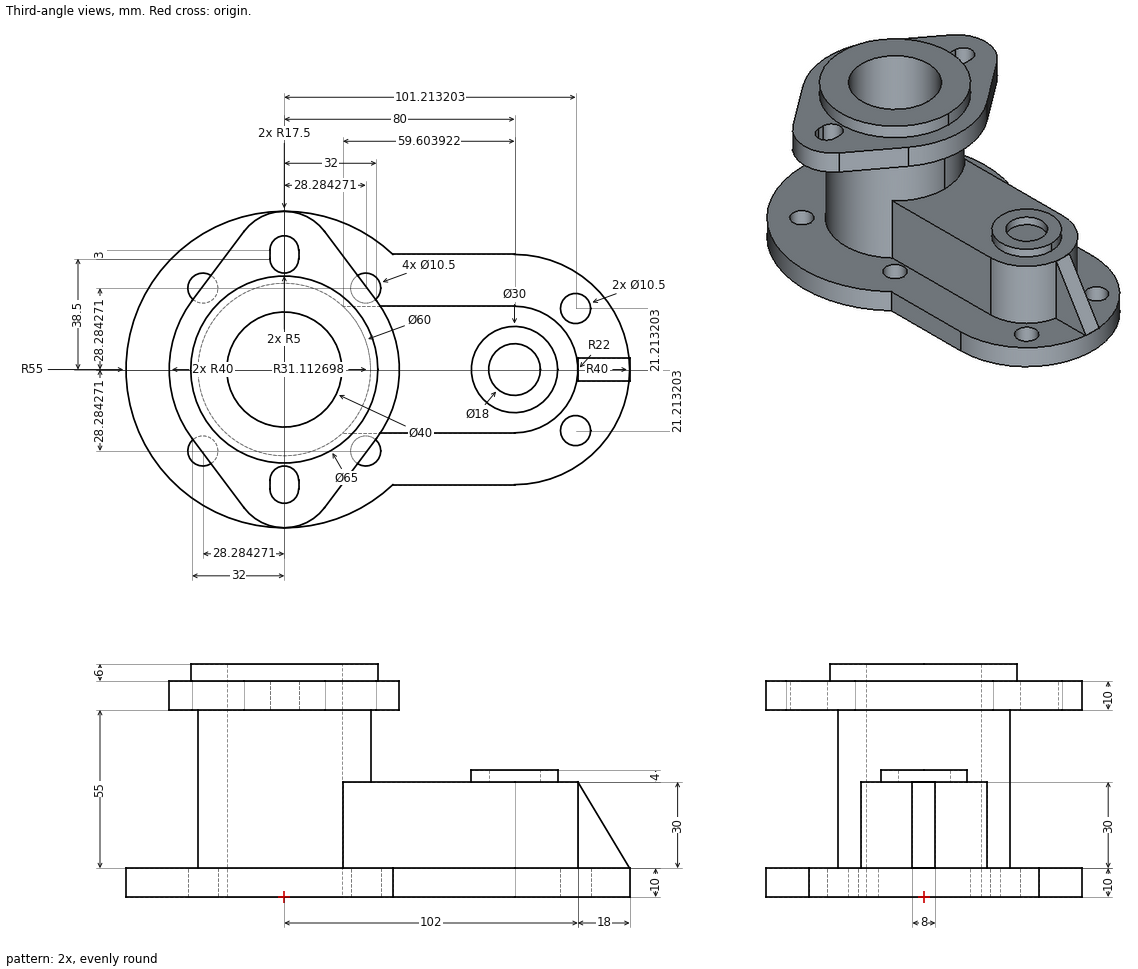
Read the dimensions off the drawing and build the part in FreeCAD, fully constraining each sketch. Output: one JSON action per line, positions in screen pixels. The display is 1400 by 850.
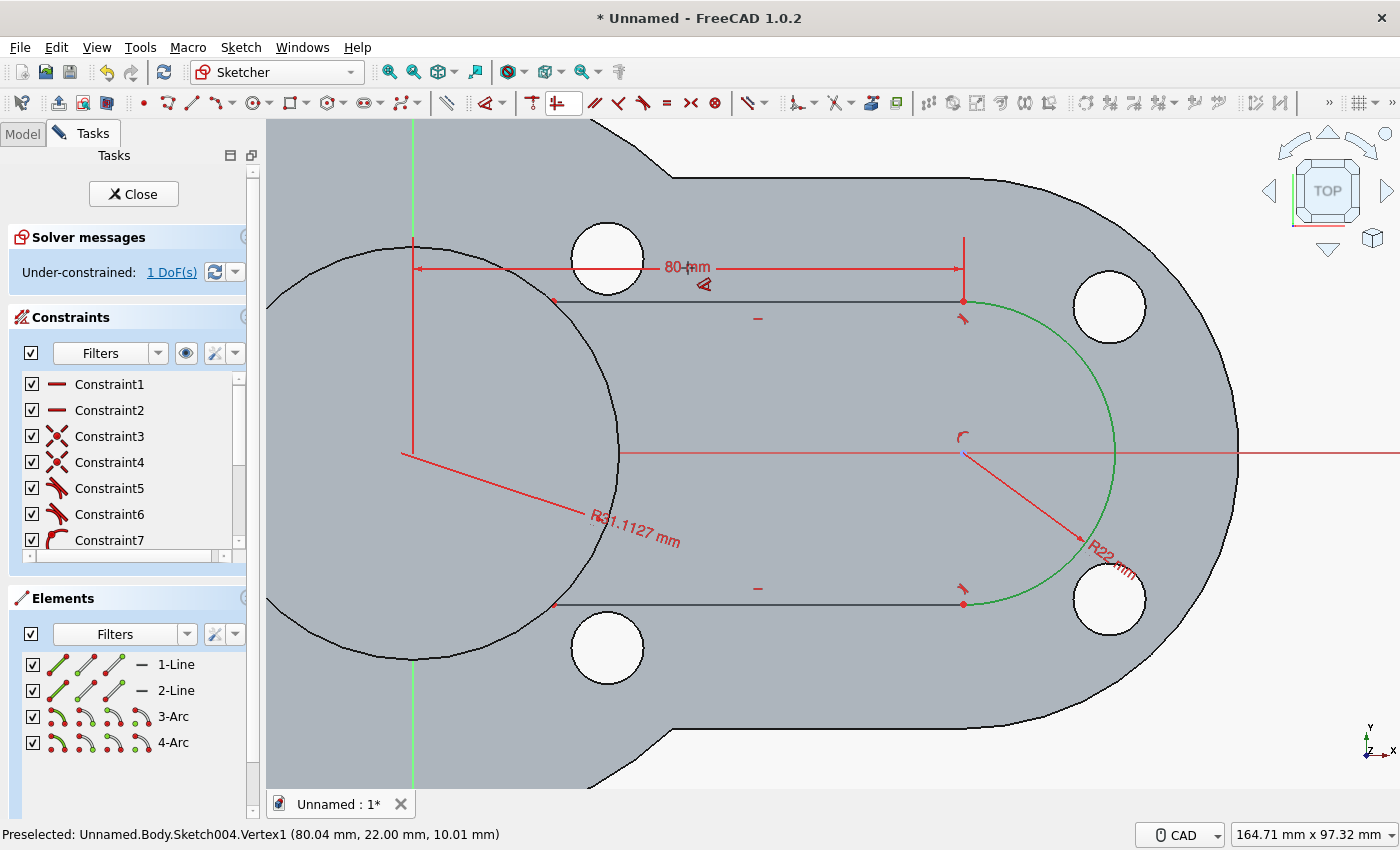
{"action": "left_click", "coordinate": [840, 302]}
{"action": "left_click", "coordinate": [853, 268]}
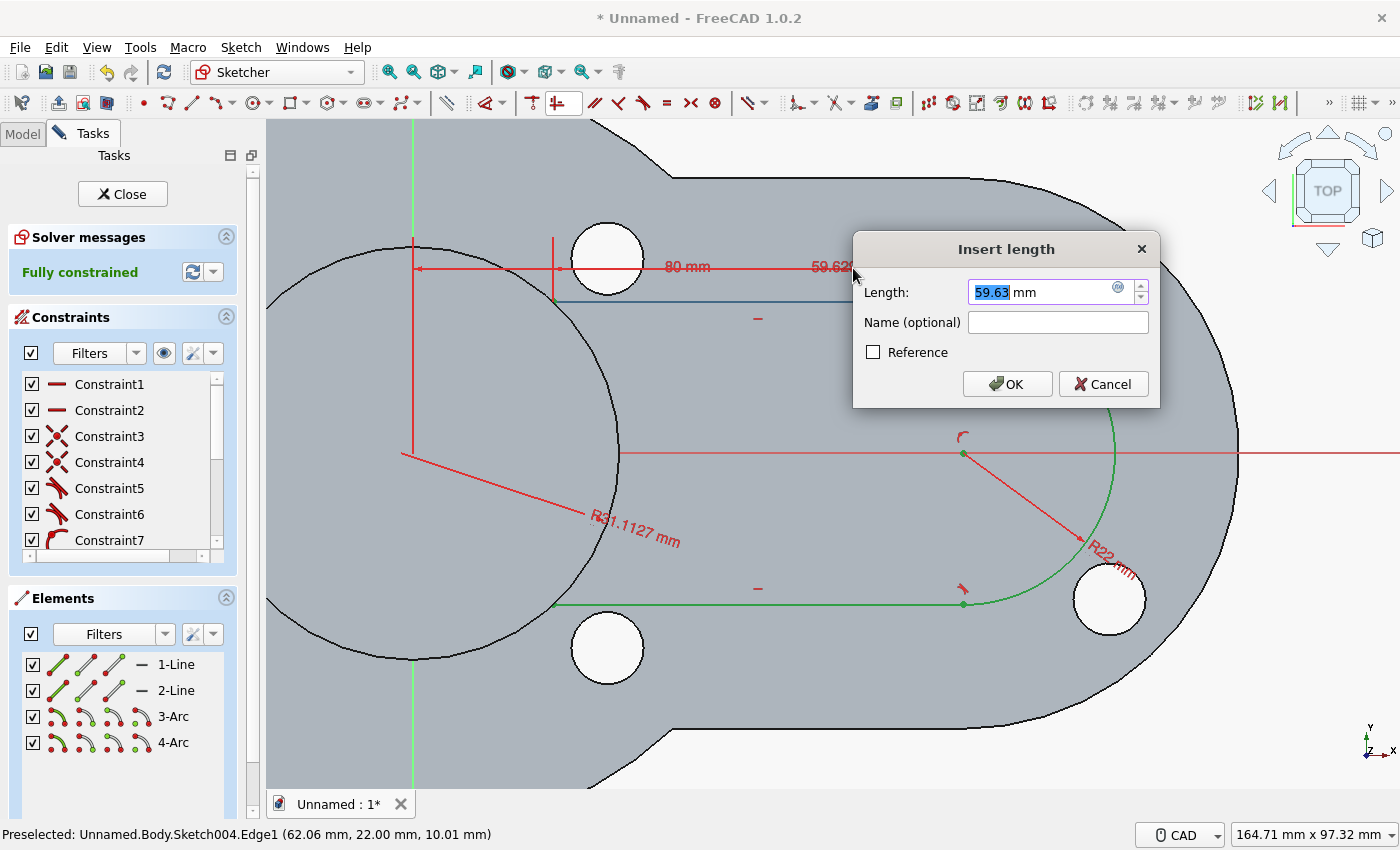
{"action": "type", "text": "59.603922"}
{"action": "key", "text": "Return"}
{"action": "key", "text": "Escape"}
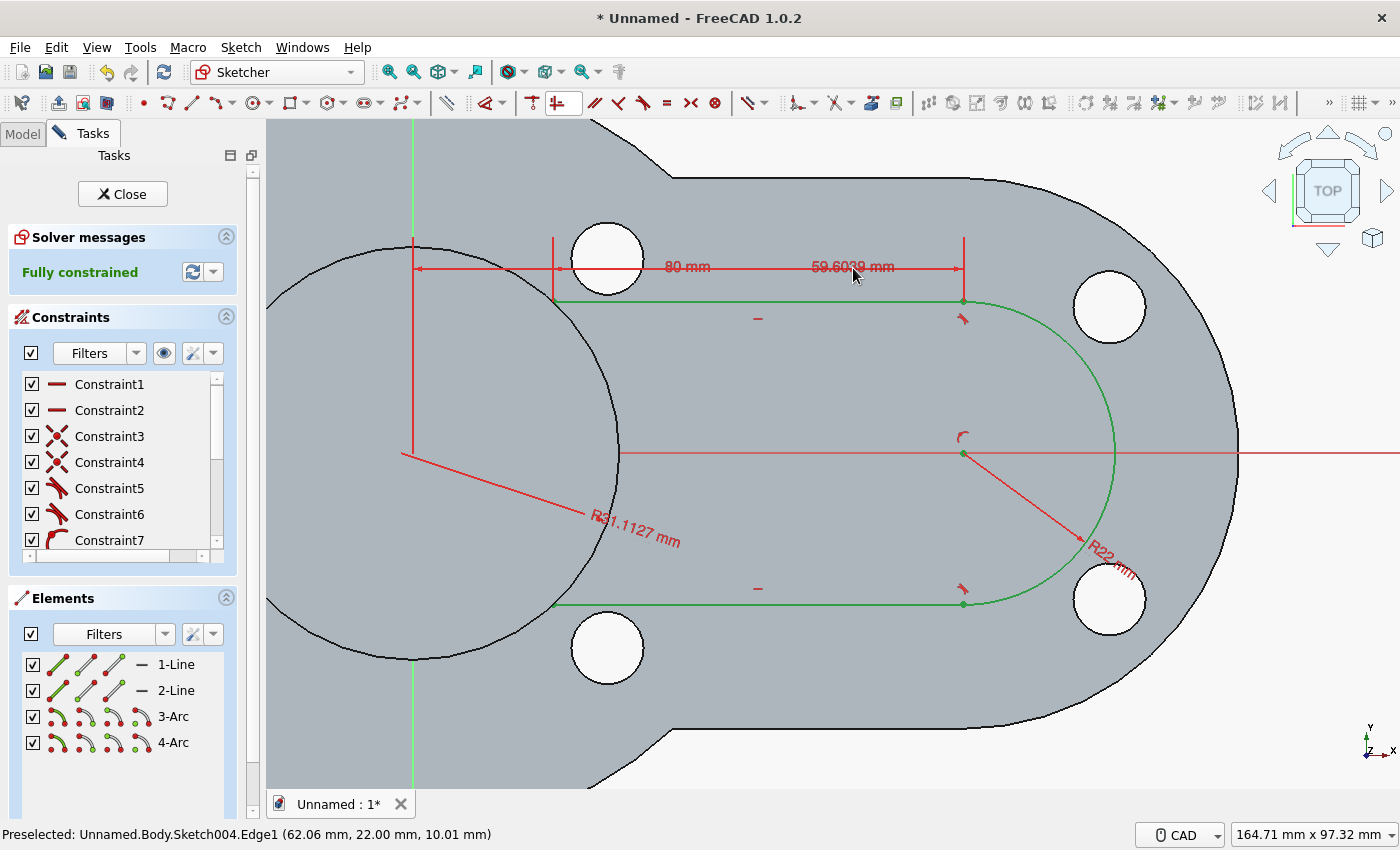
{"action": "left_click", "coordinate": [123, 194]}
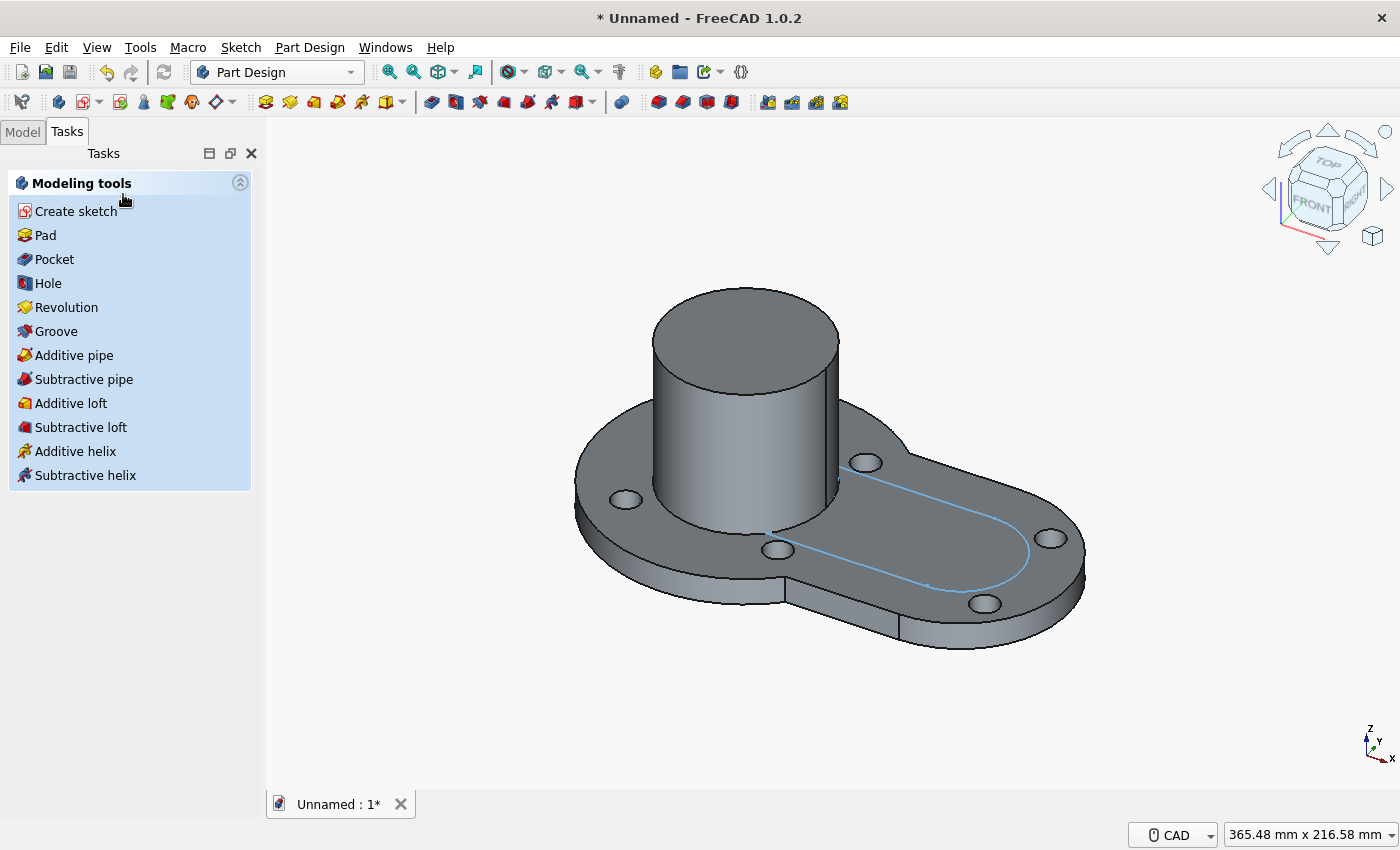
{"action": "left_click", "coordinate": [266, 102]}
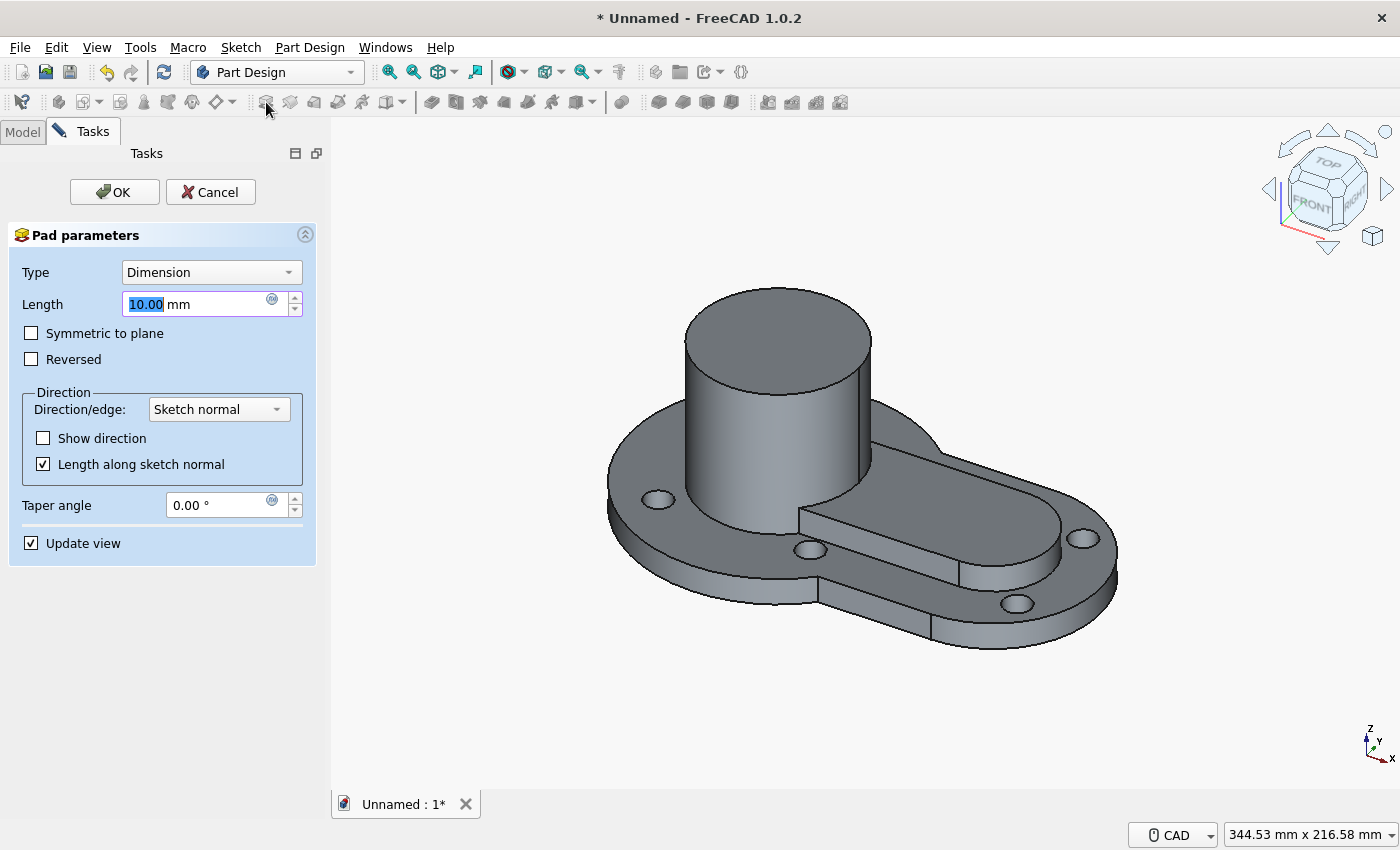
{"action": "type", "text": "30"}
{"action": "key", "text": "Tab"}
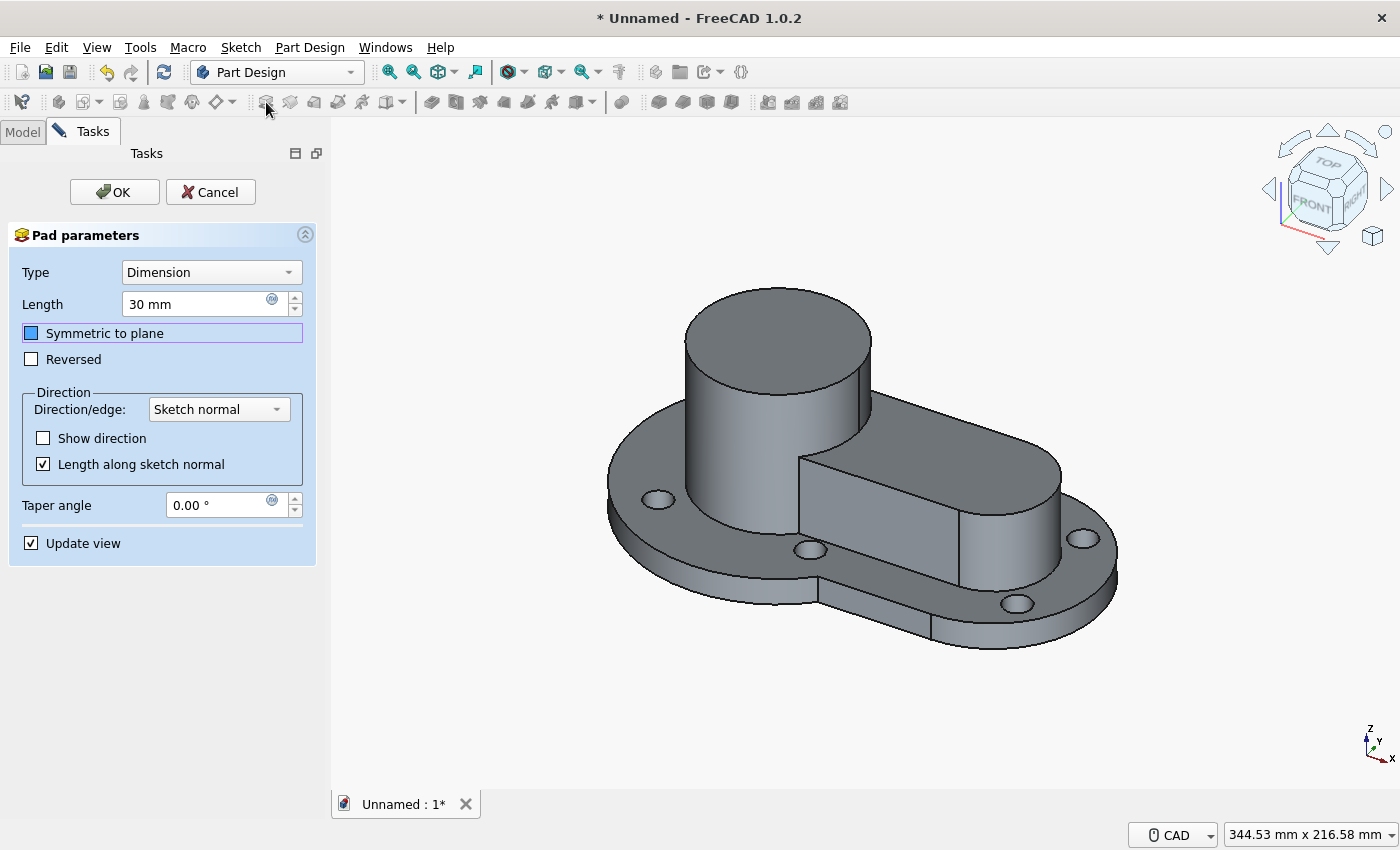
{"action": "left_click", "coordinate": [115, 192]}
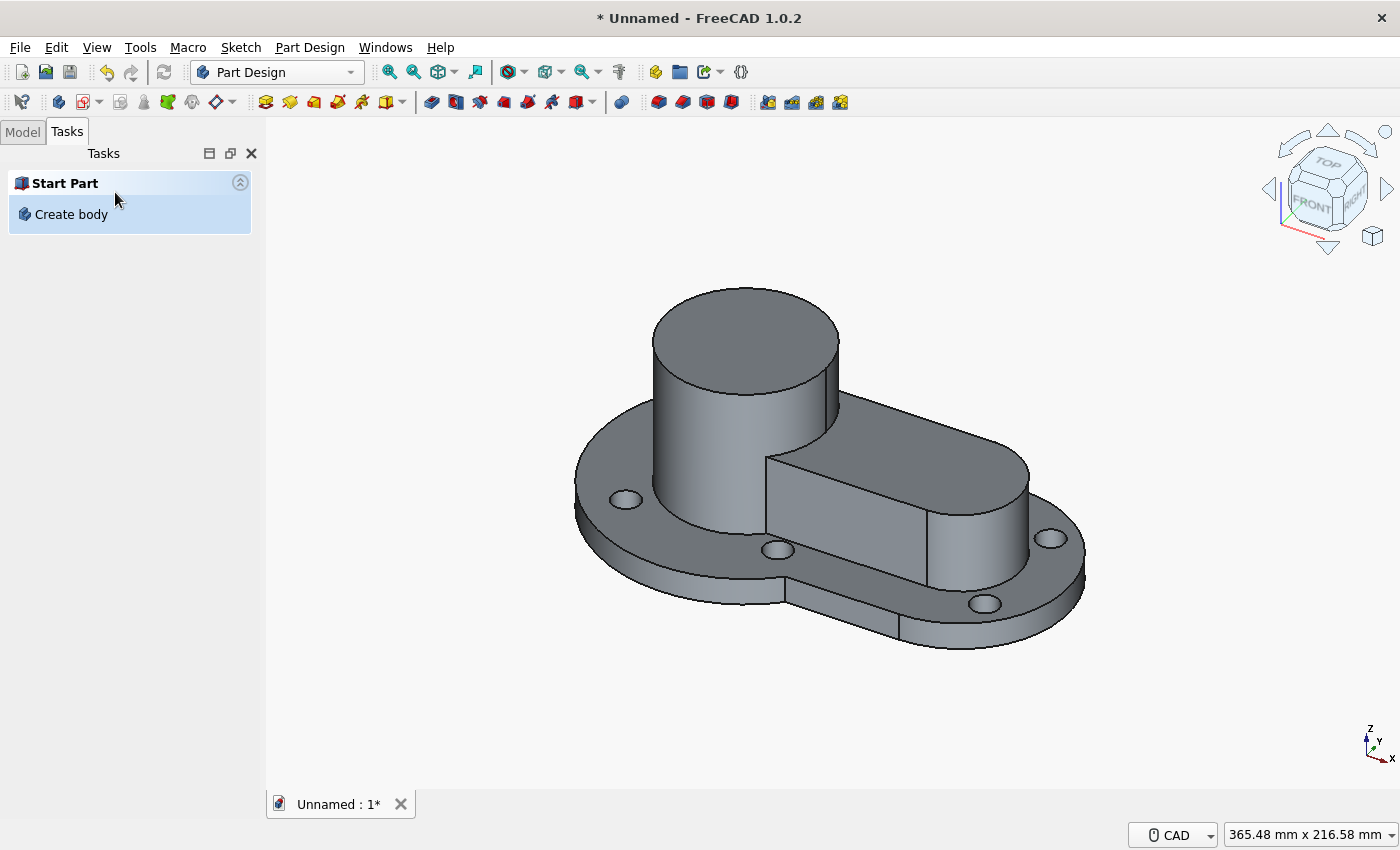
{"action": "left_click", "coordinate": [942, 469]}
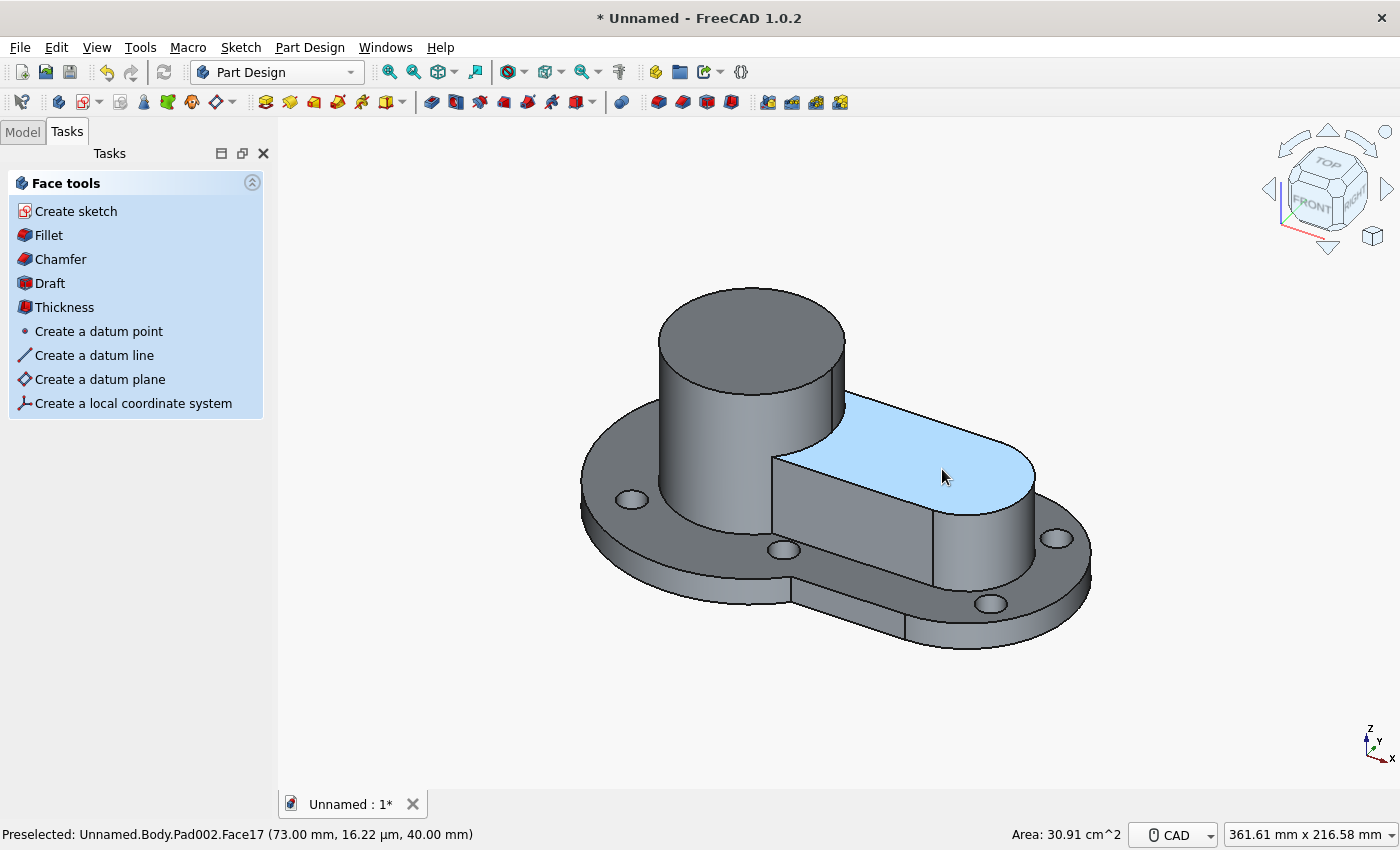
{"action": "left_click", "coordinate": [84, 102]}